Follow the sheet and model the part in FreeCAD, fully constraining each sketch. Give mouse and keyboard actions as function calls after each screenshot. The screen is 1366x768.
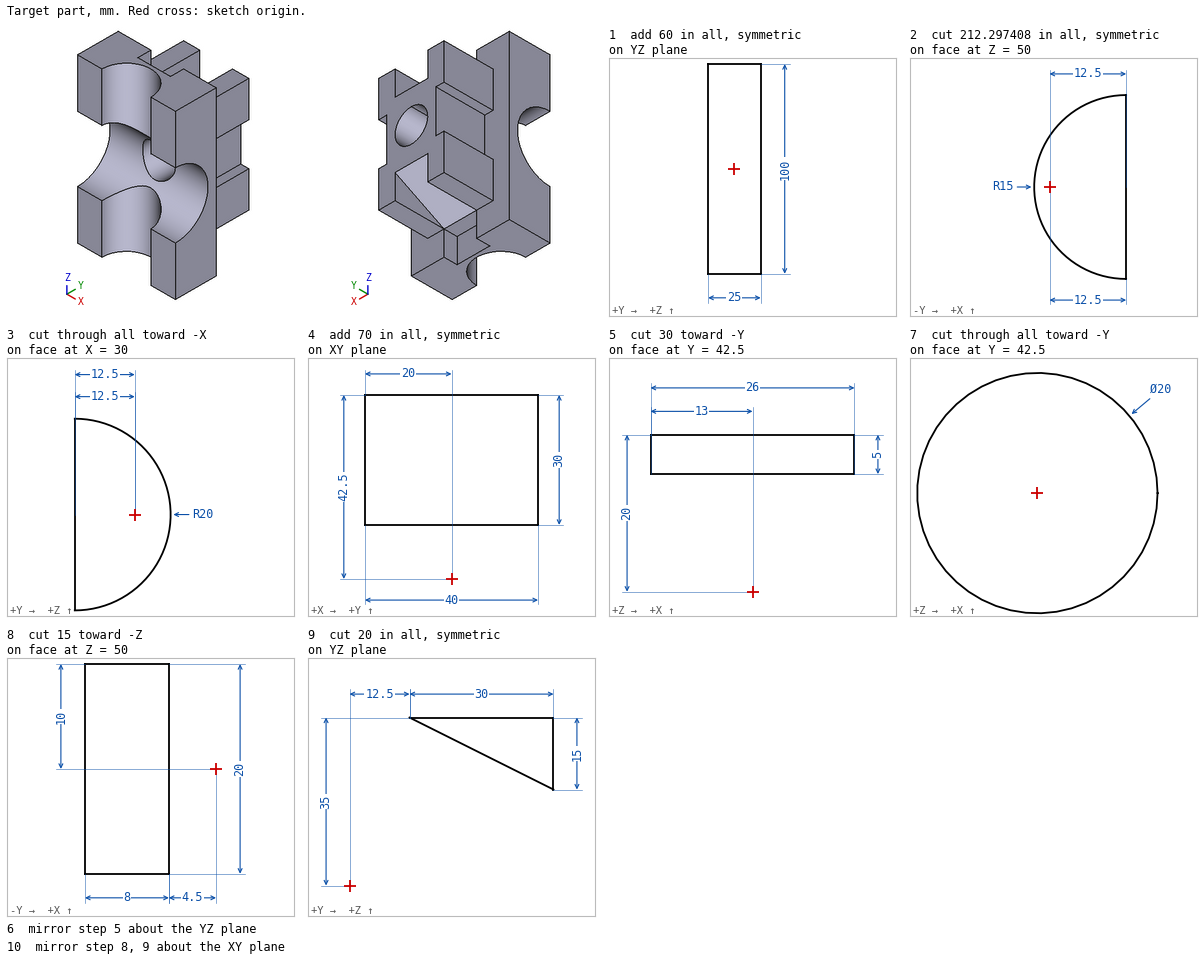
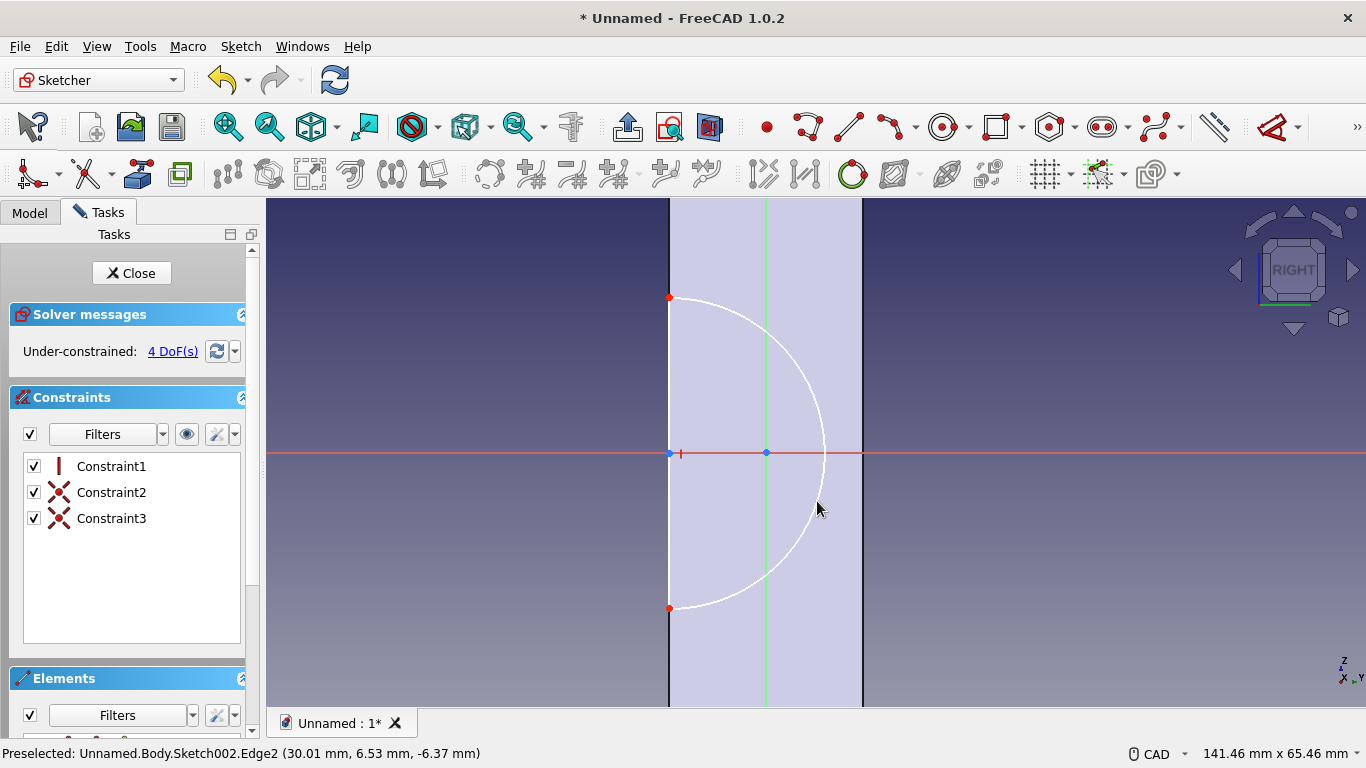
click(669, 453)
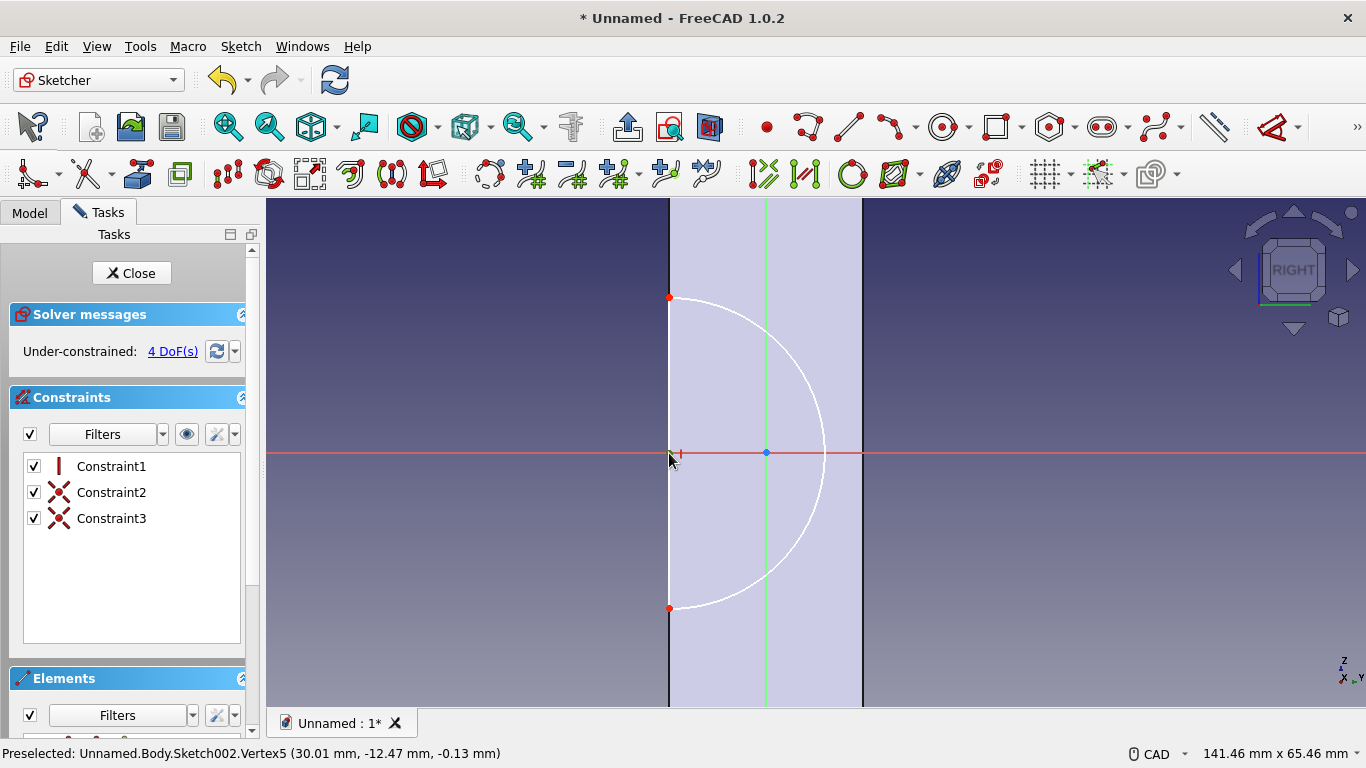
click(359, 452)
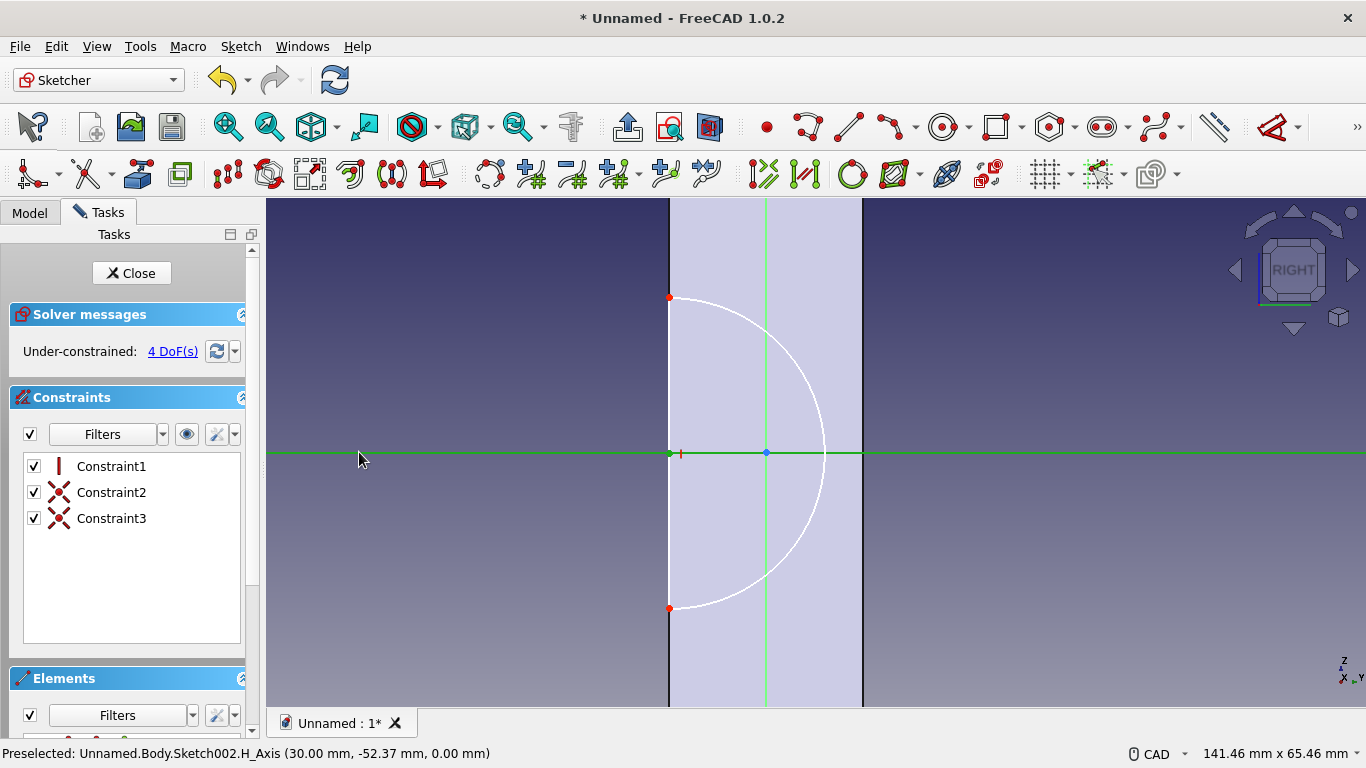
key(c)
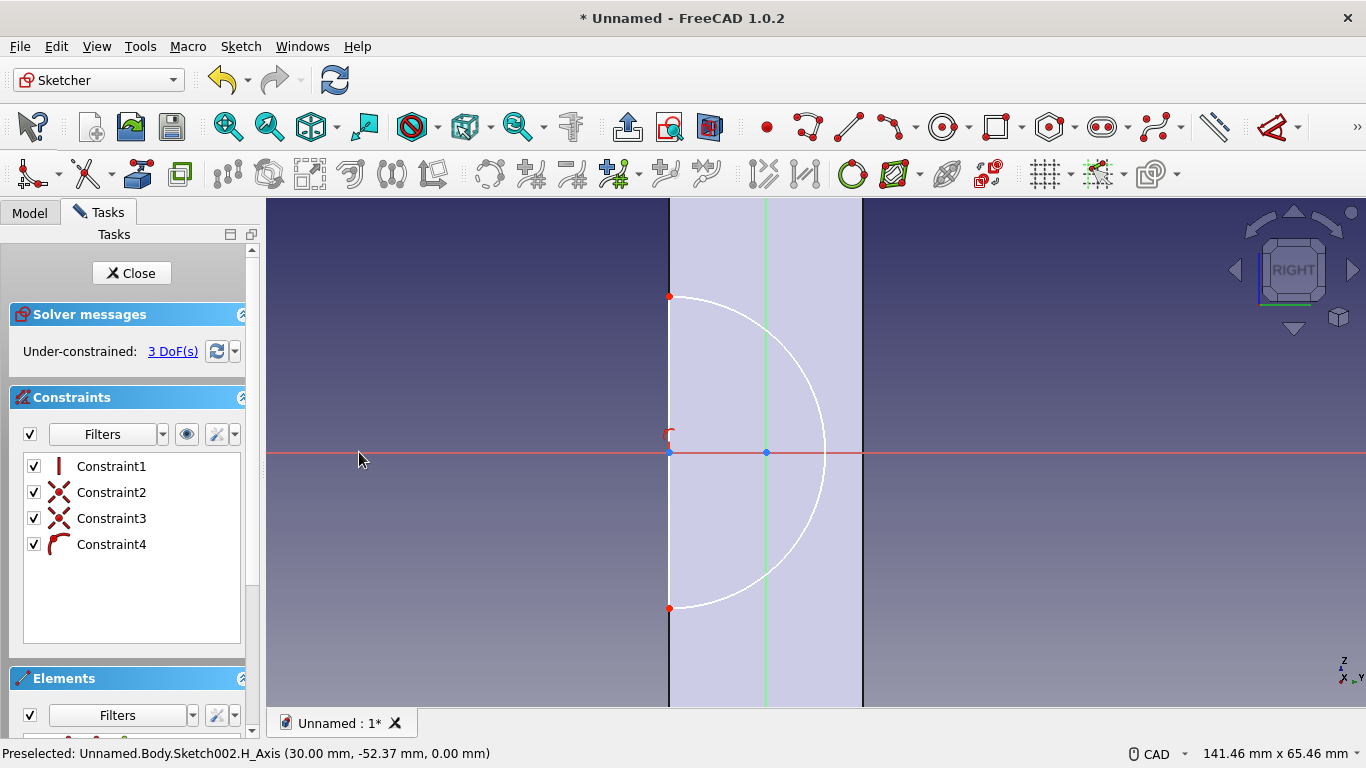
click(795, 544)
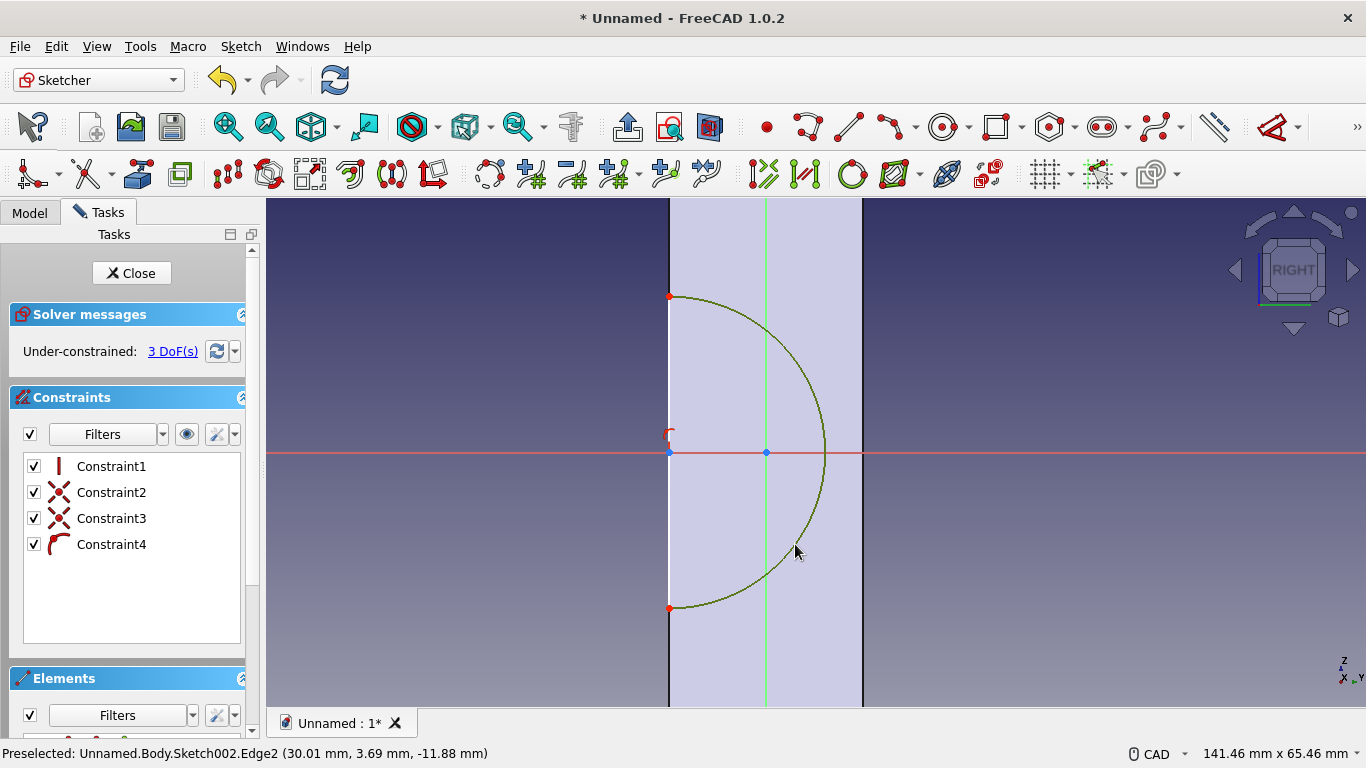
click(1298, 128)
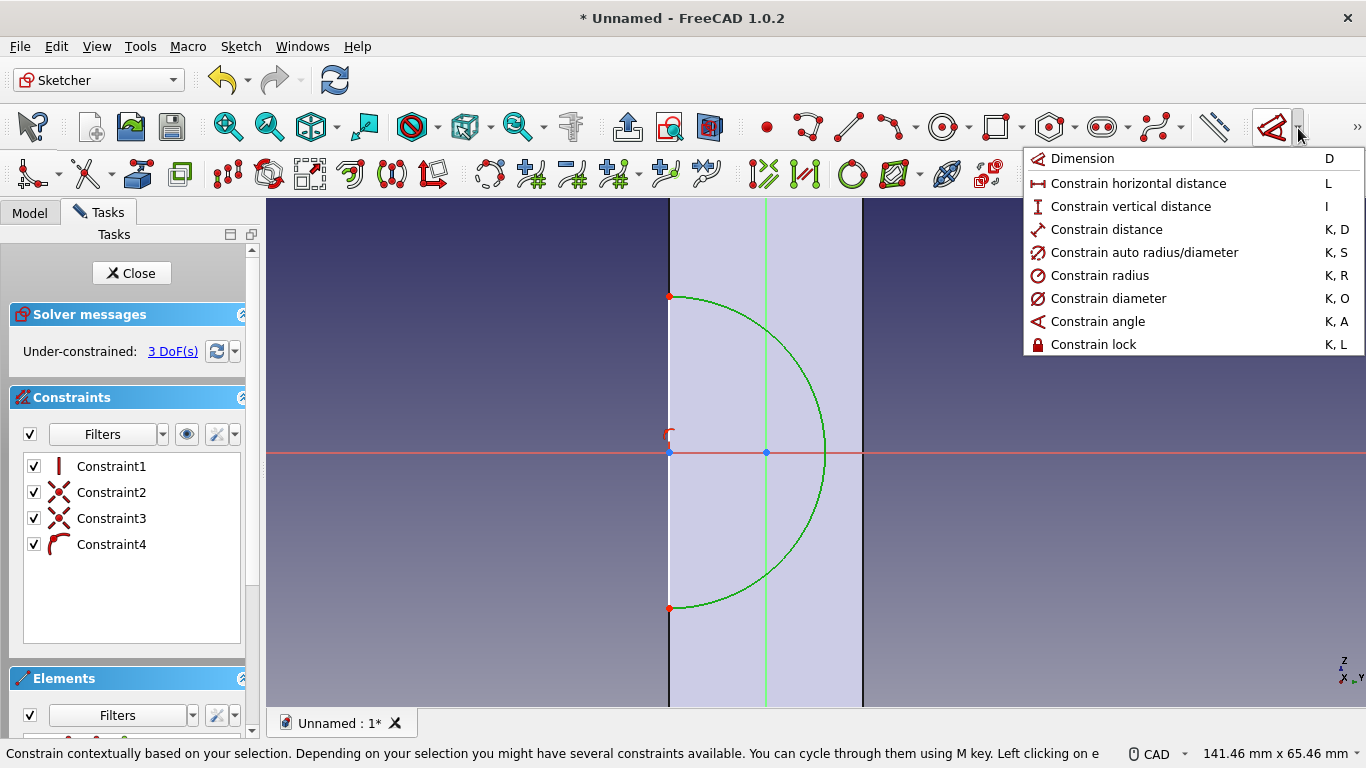
click(1194, 276)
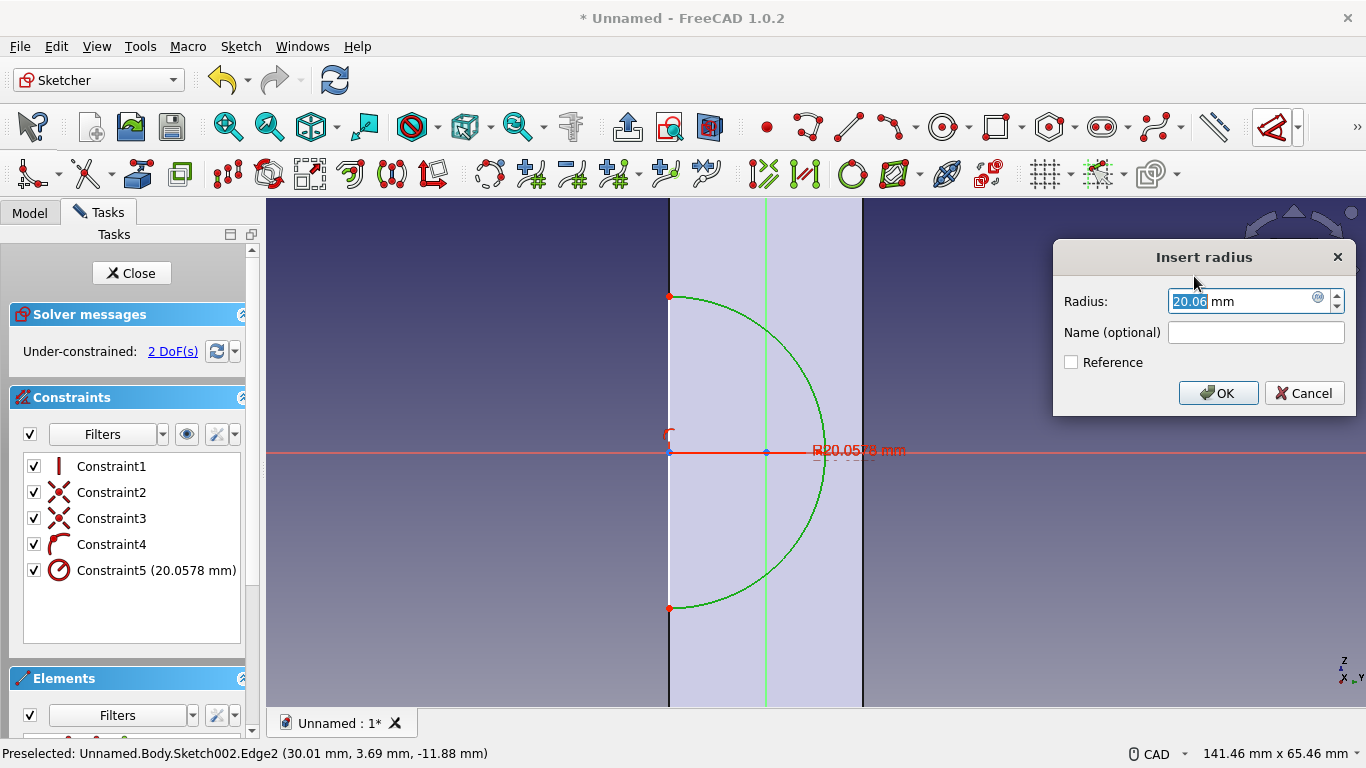
text(20)
key(Return)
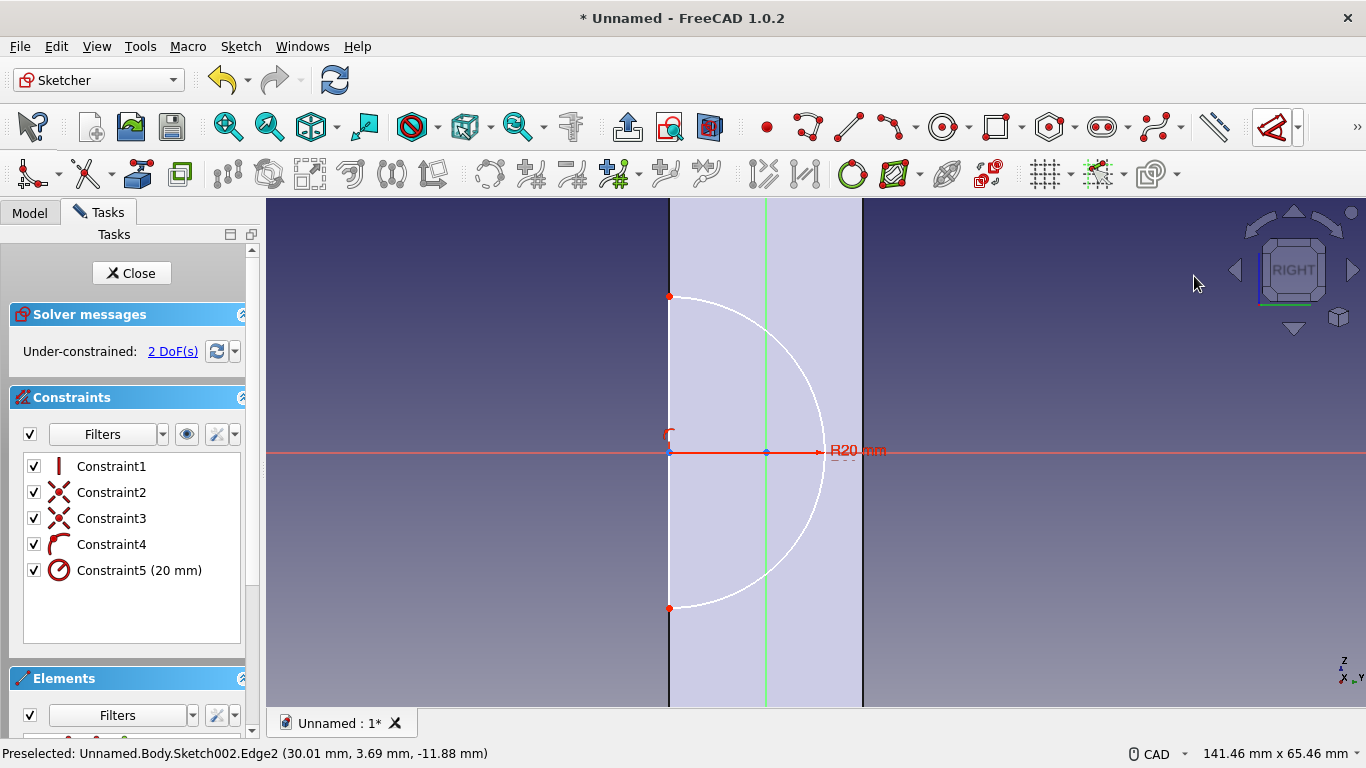
click(669, 297)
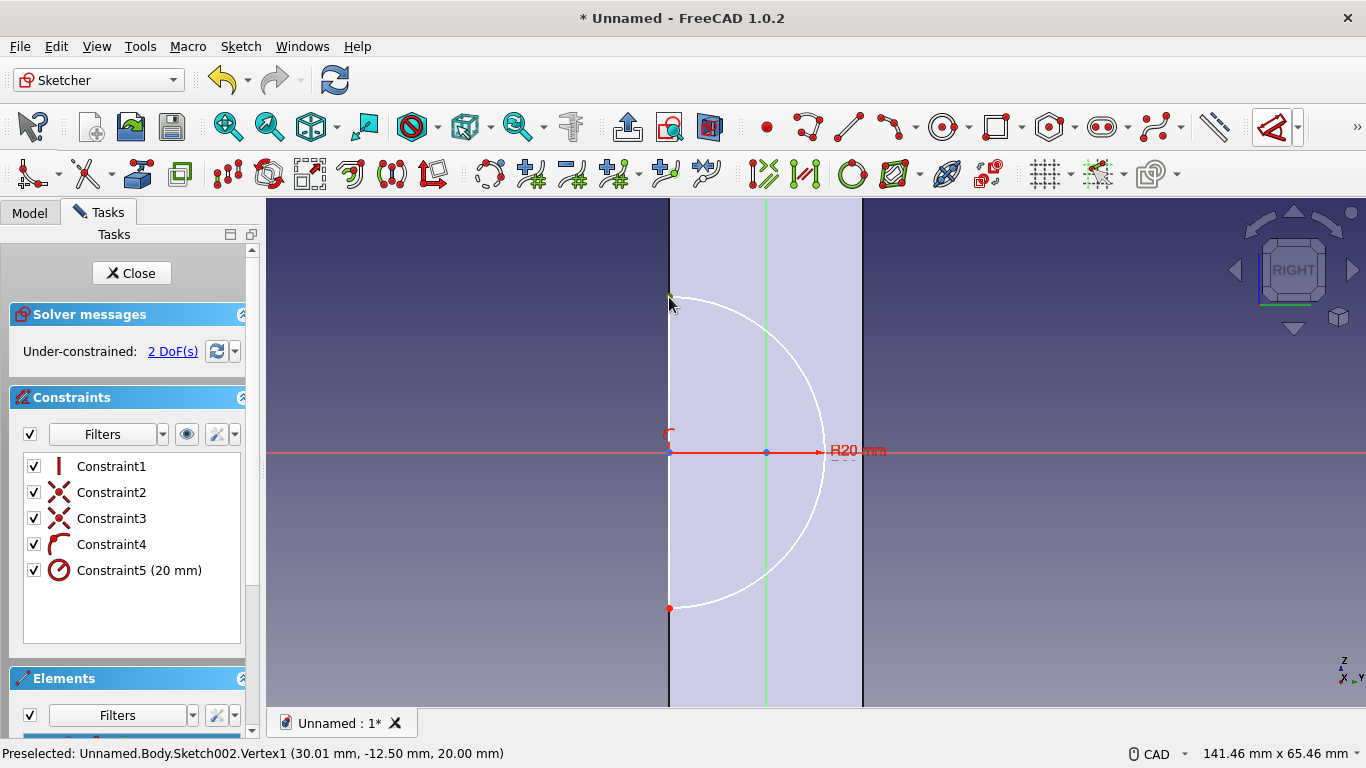
key(l)